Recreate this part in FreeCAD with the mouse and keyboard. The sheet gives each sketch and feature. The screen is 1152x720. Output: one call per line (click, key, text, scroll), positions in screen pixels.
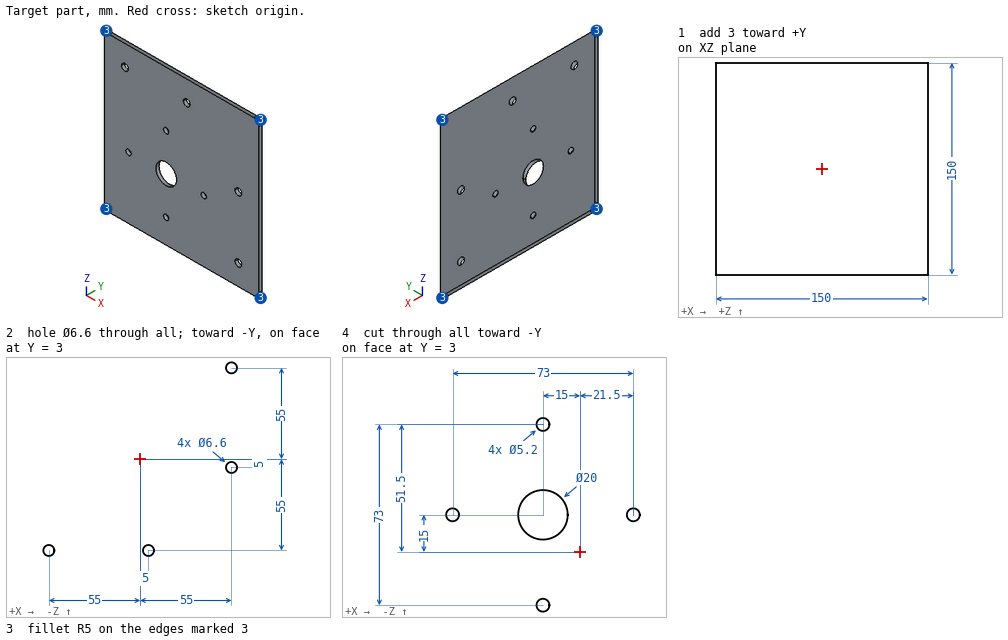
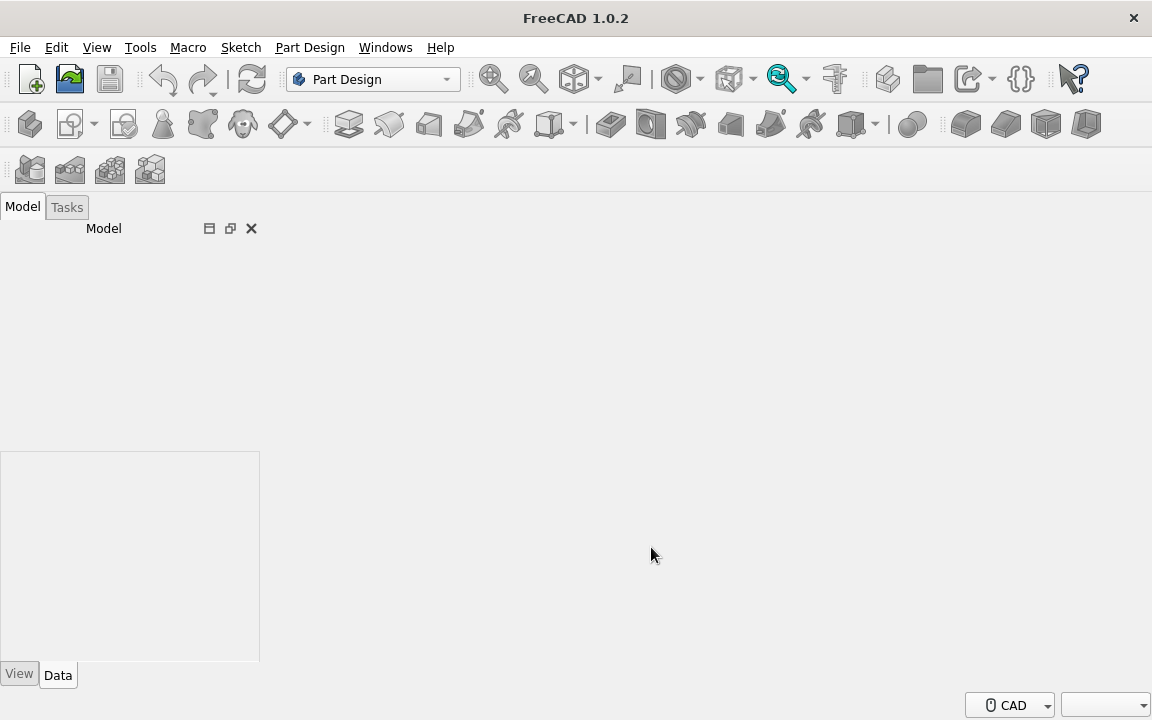
click(30, 80)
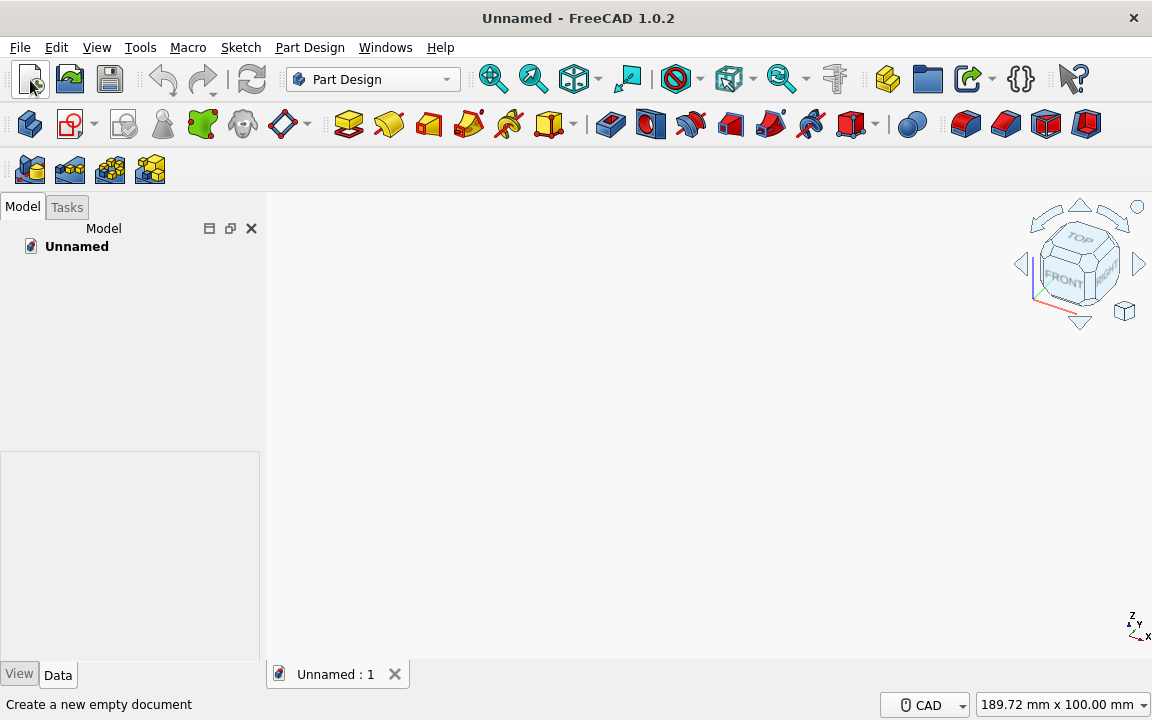
click(70, 124)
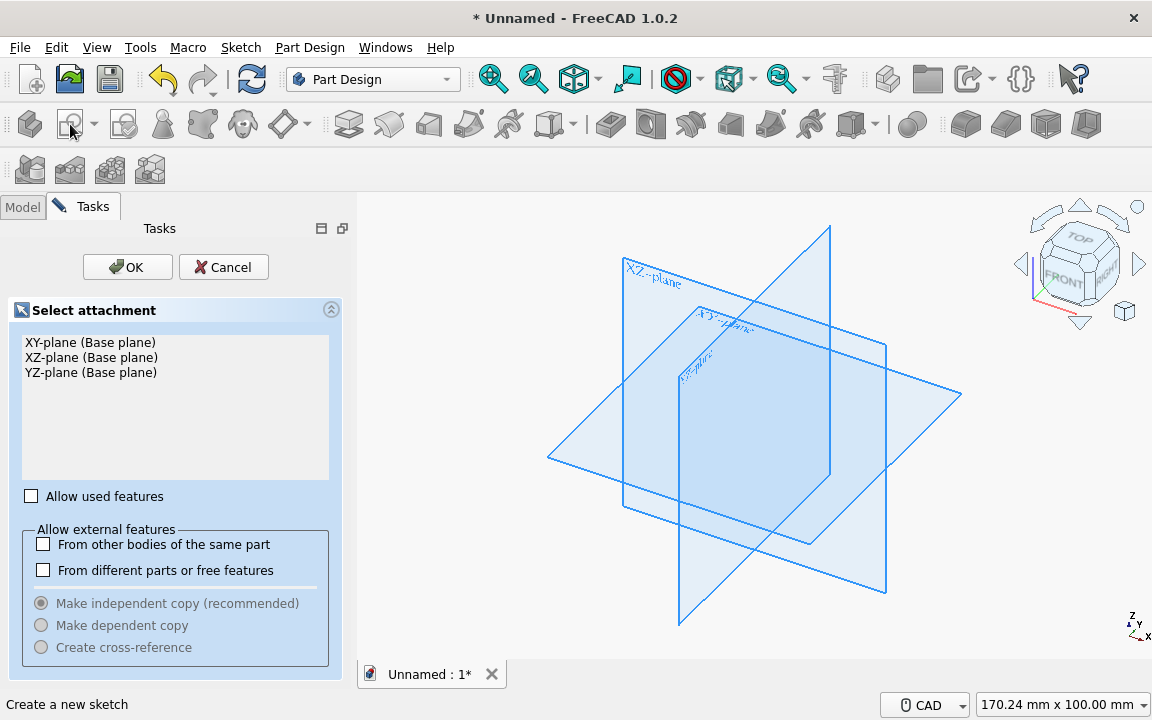
click(82, 358)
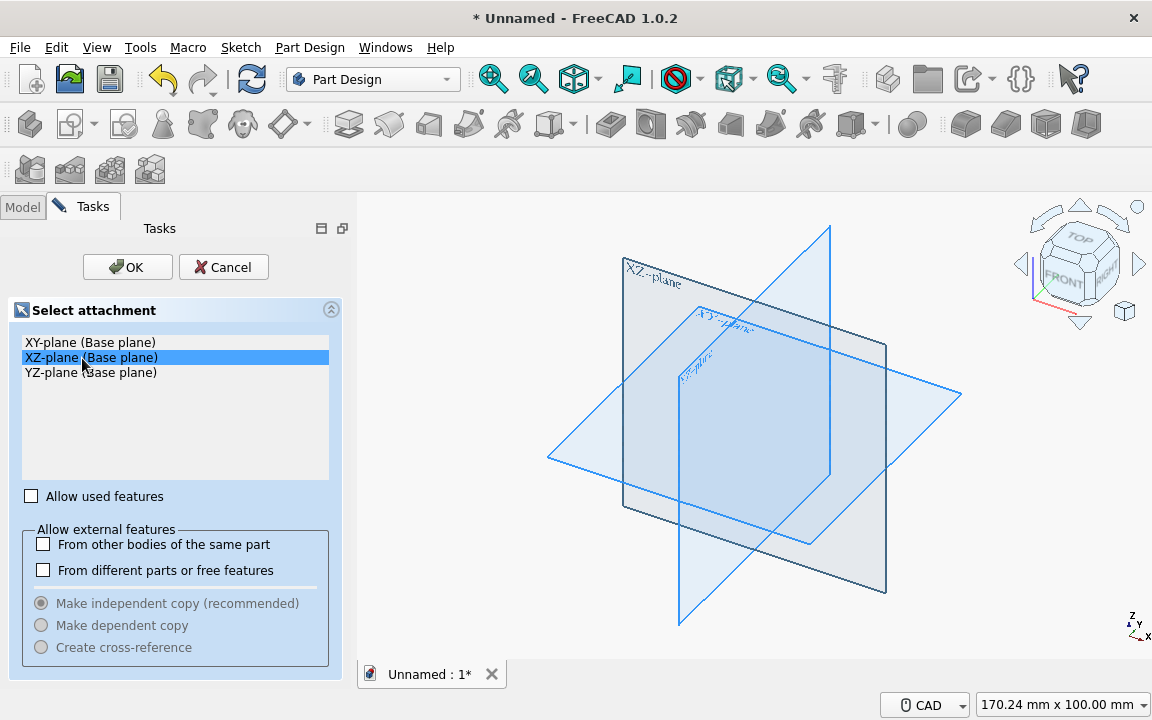
click(128, 267)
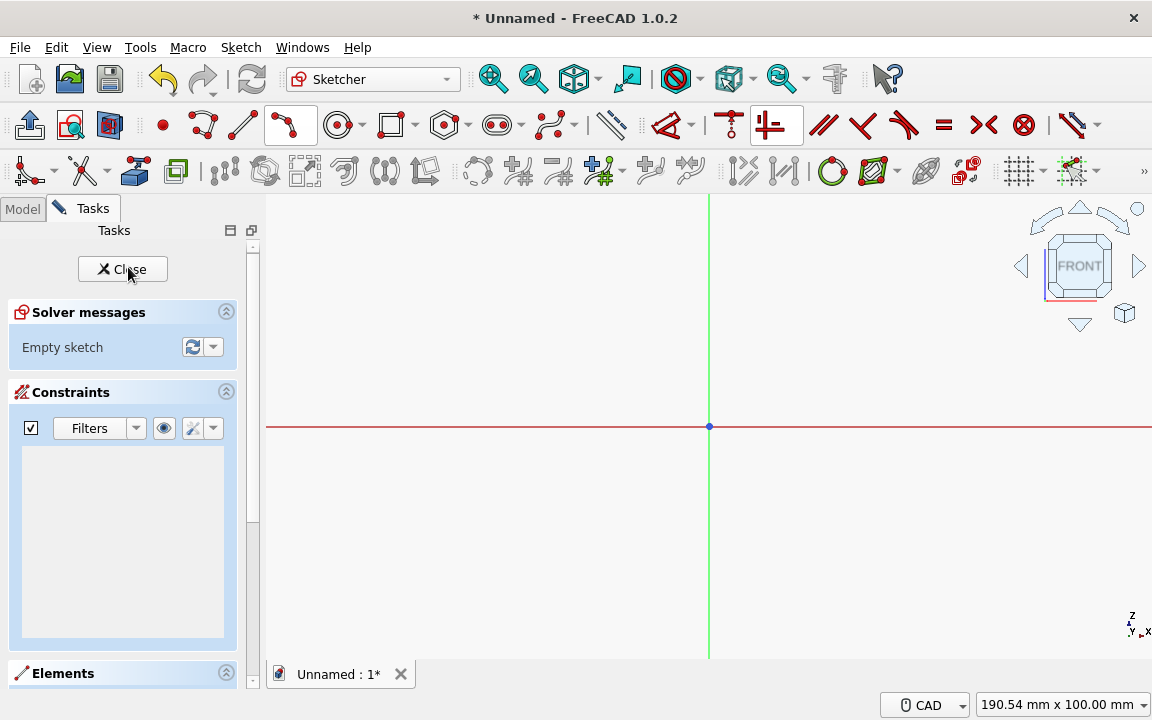
scroll(585, 426, down, 4)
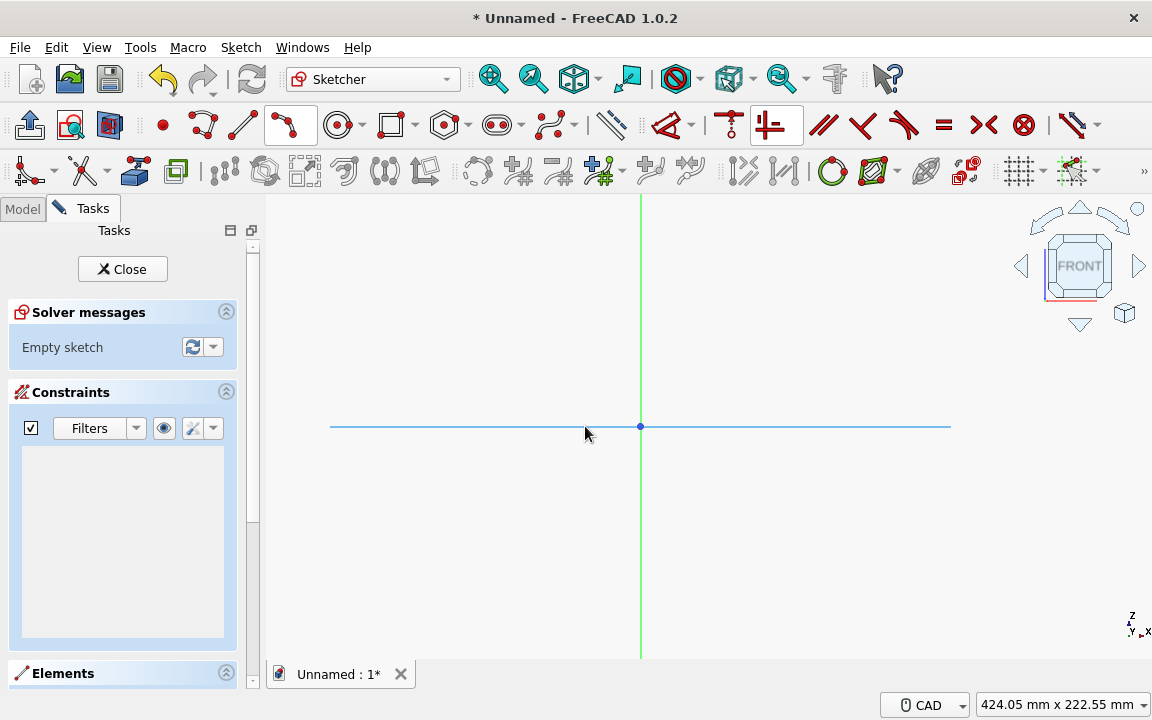
click(418, 126)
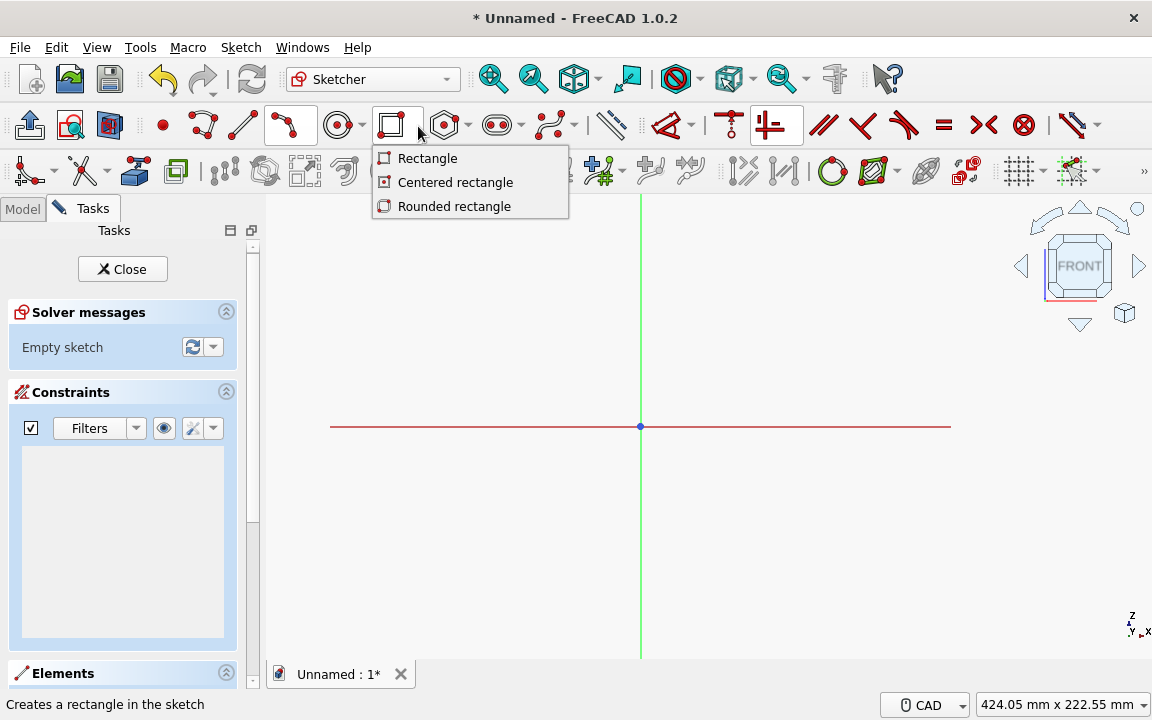
click(470, 182)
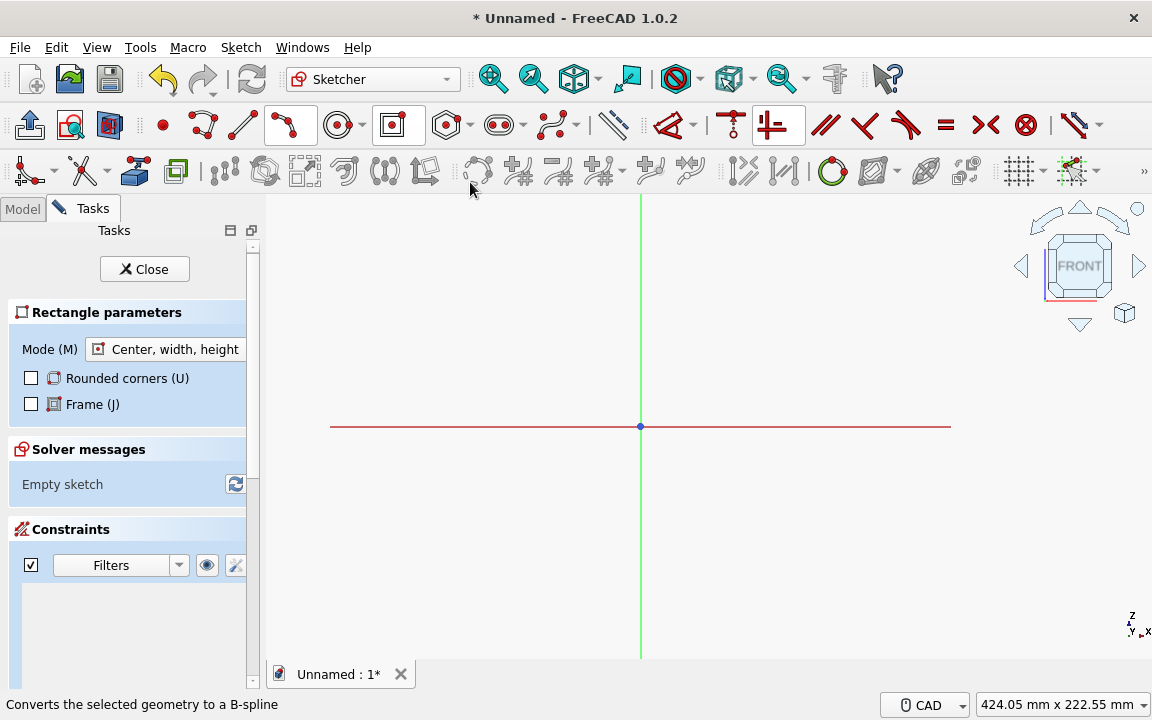
click(641, 426)
click(798, 270)
key(Escape)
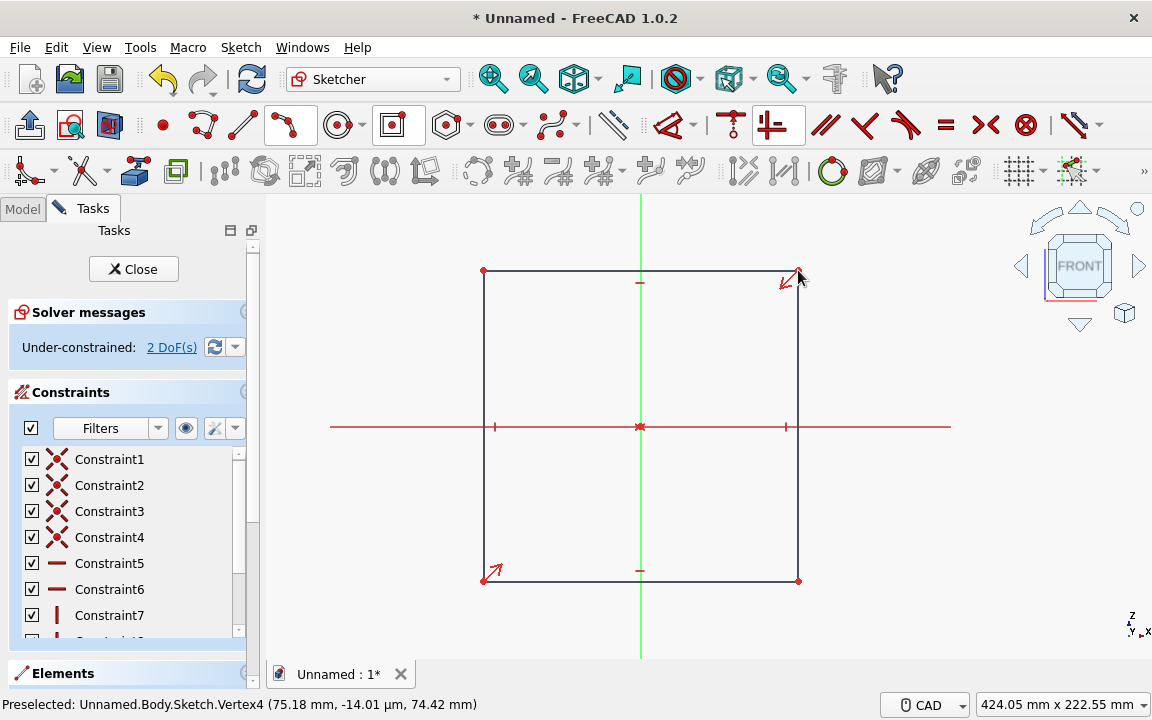
click(668, 126)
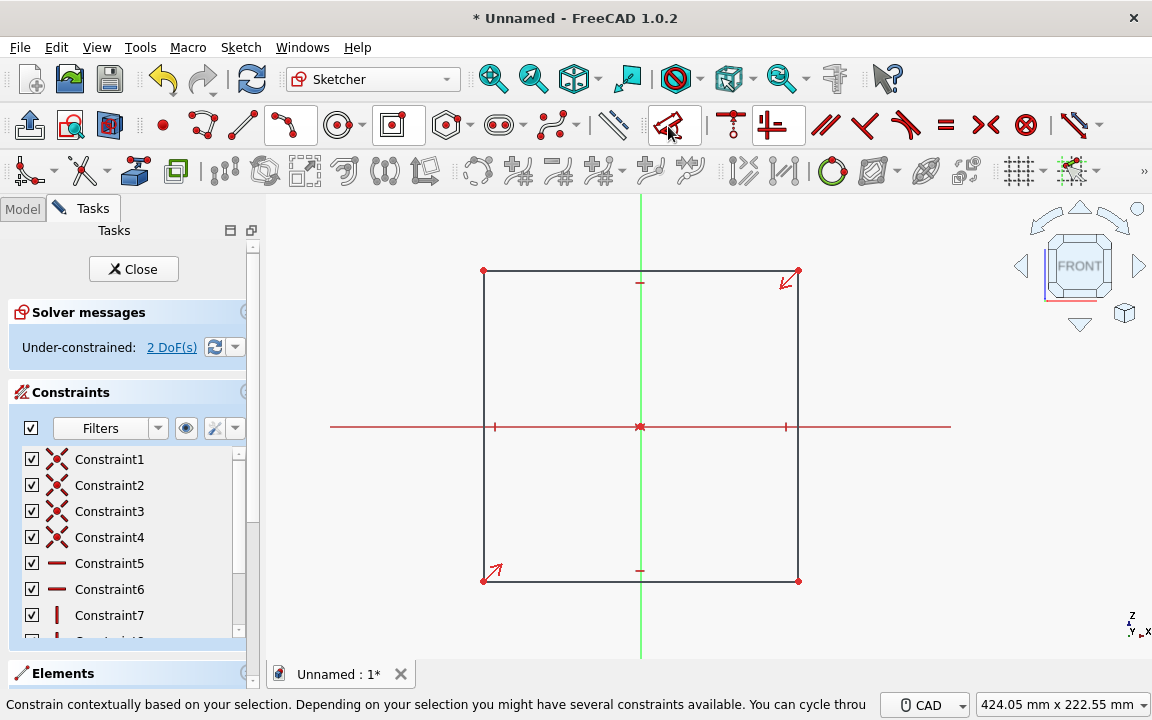
click(578, 582)
click(569, 616)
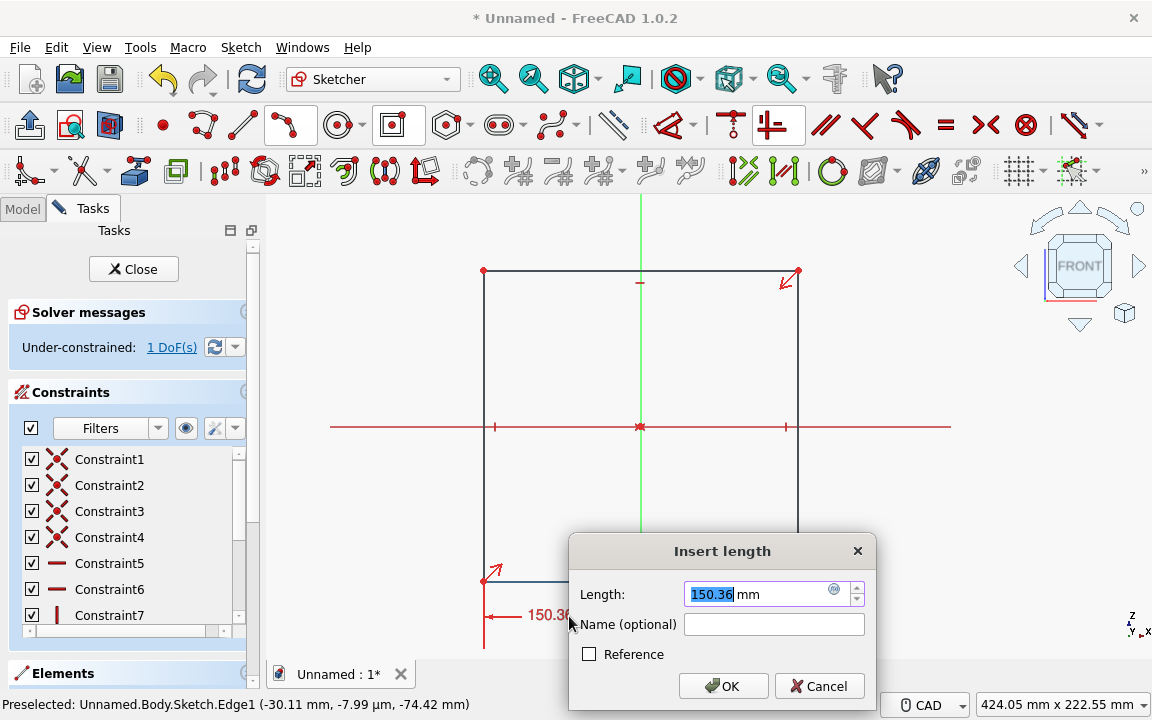
text(150)
key(Return)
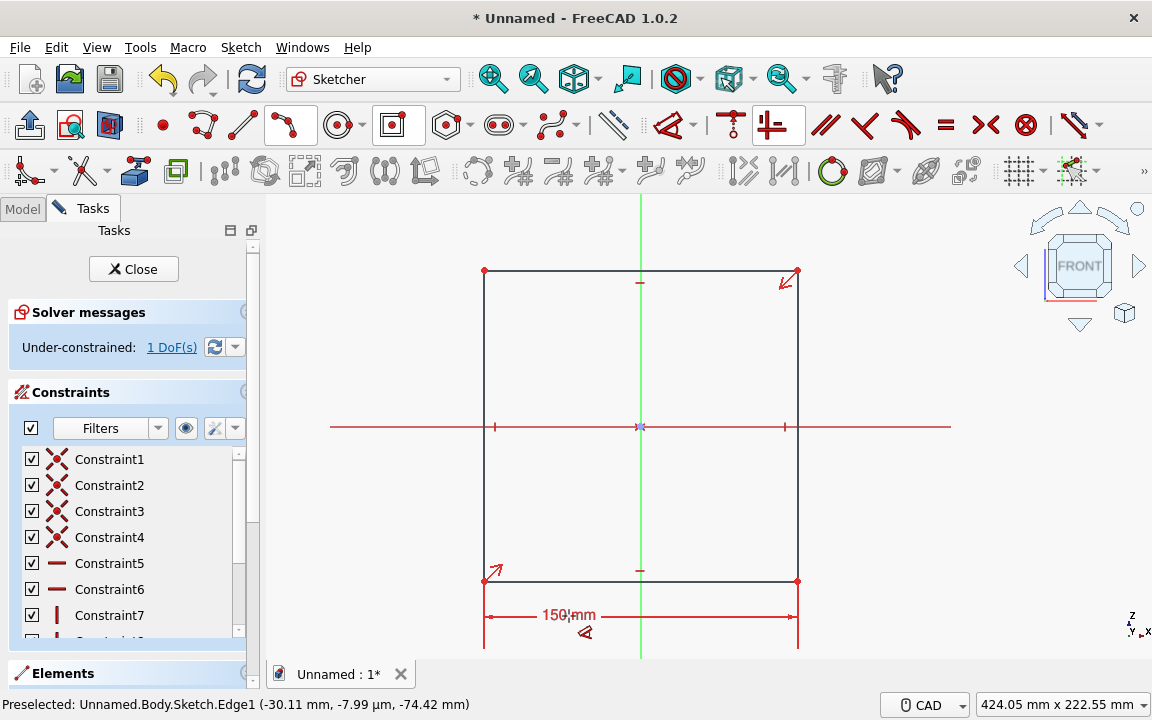
click(798, 489)
click(832, 355)